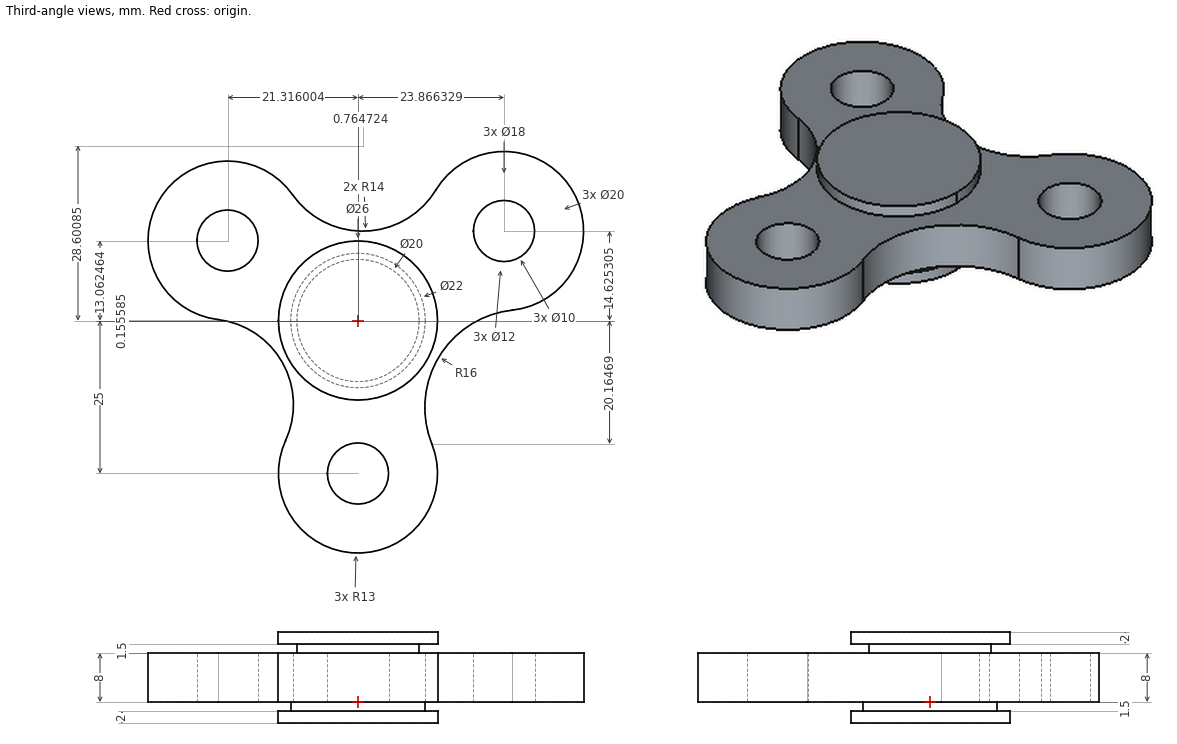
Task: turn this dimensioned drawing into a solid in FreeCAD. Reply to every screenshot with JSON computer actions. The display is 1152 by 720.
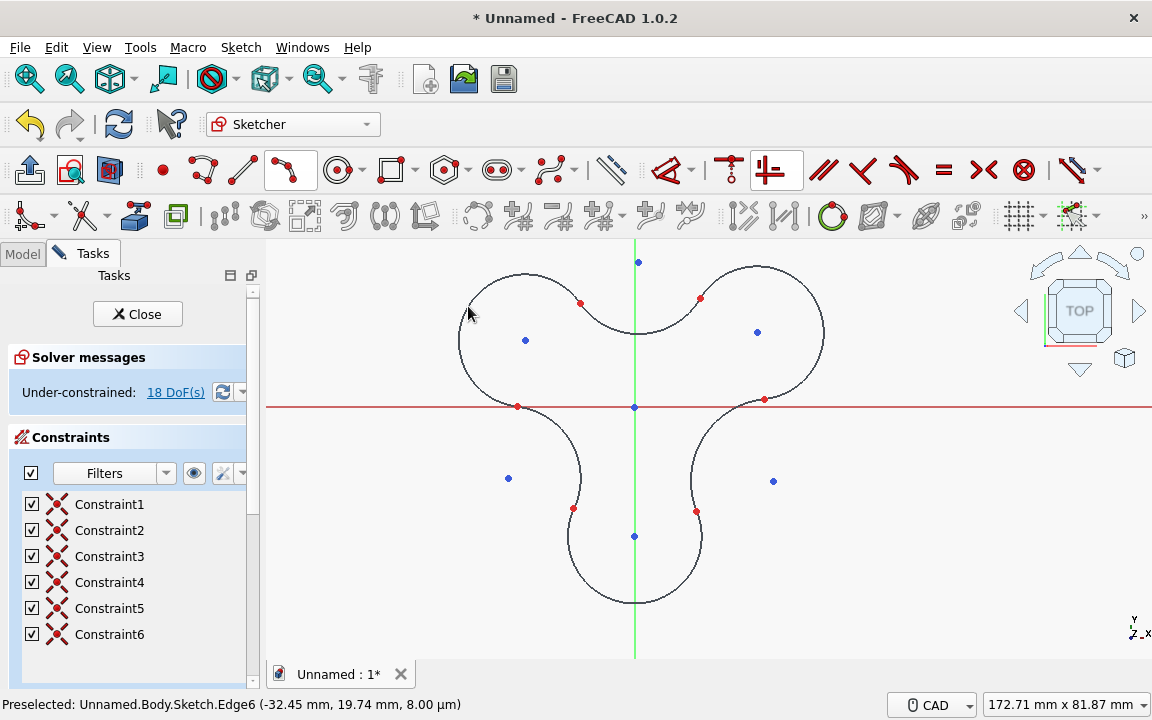
{"action": "left_click", "coordinate": [580, 469]}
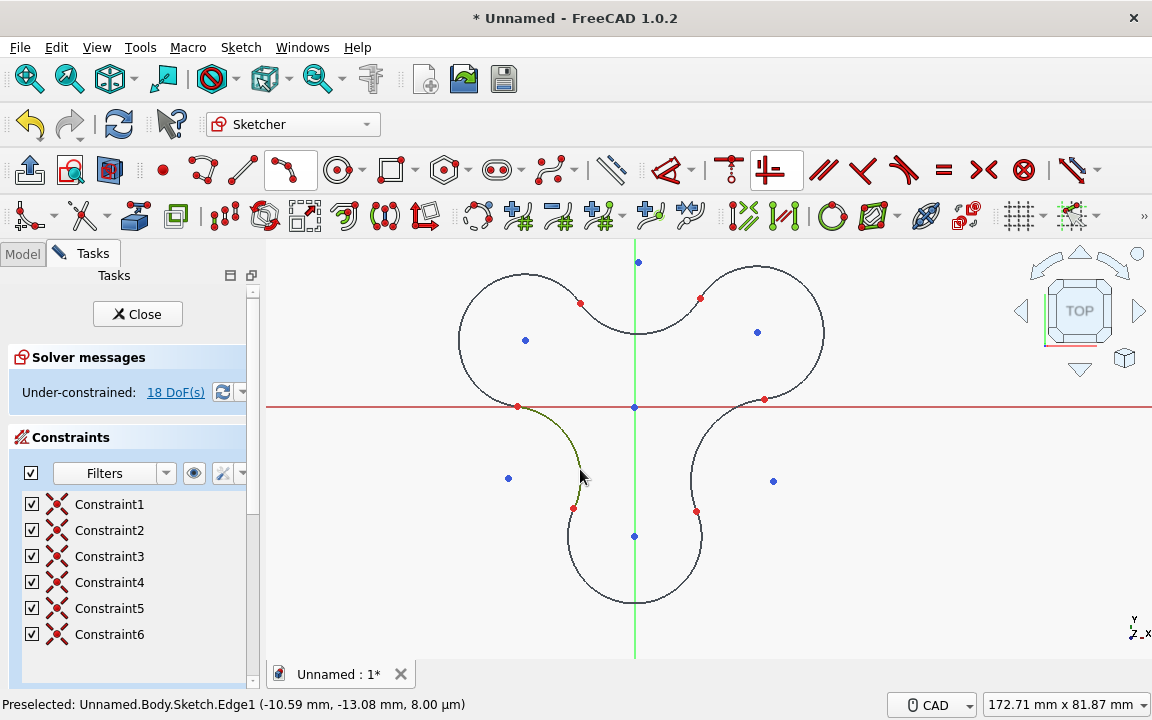
{"action": "left_click", "coordinate": [586, 583]}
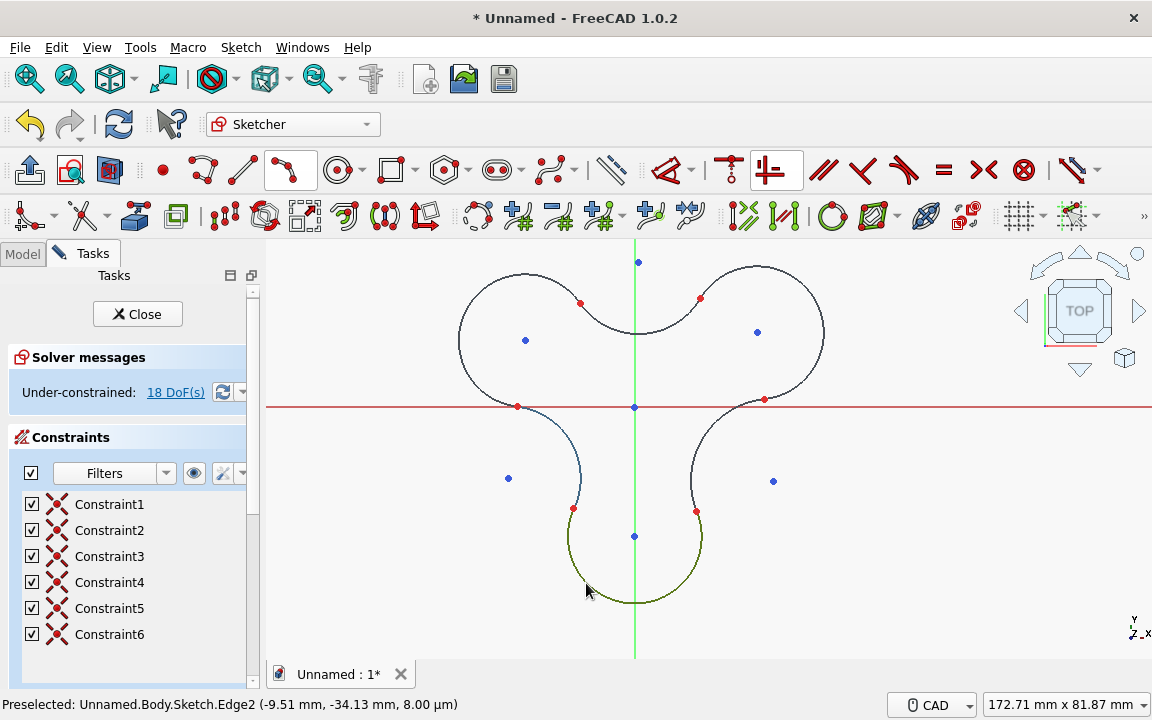
{"action": "left_click", "coordinate": [904, 170]}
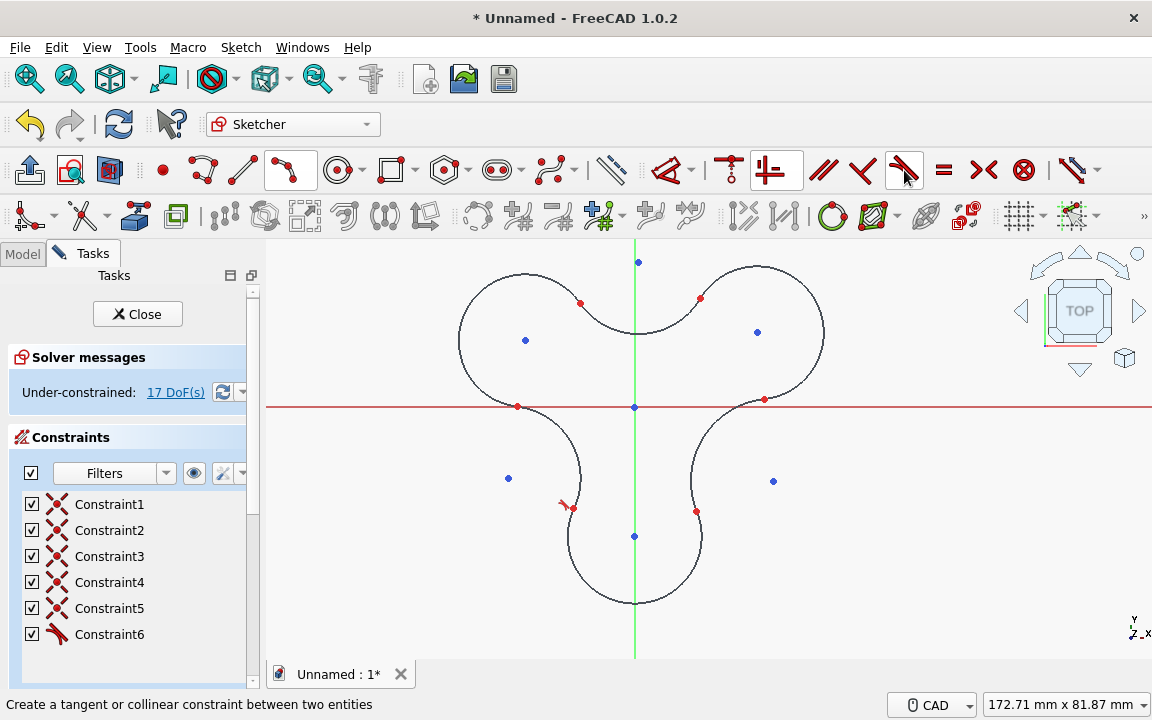
{"action": "left_click", "coordinate": [580, 469]}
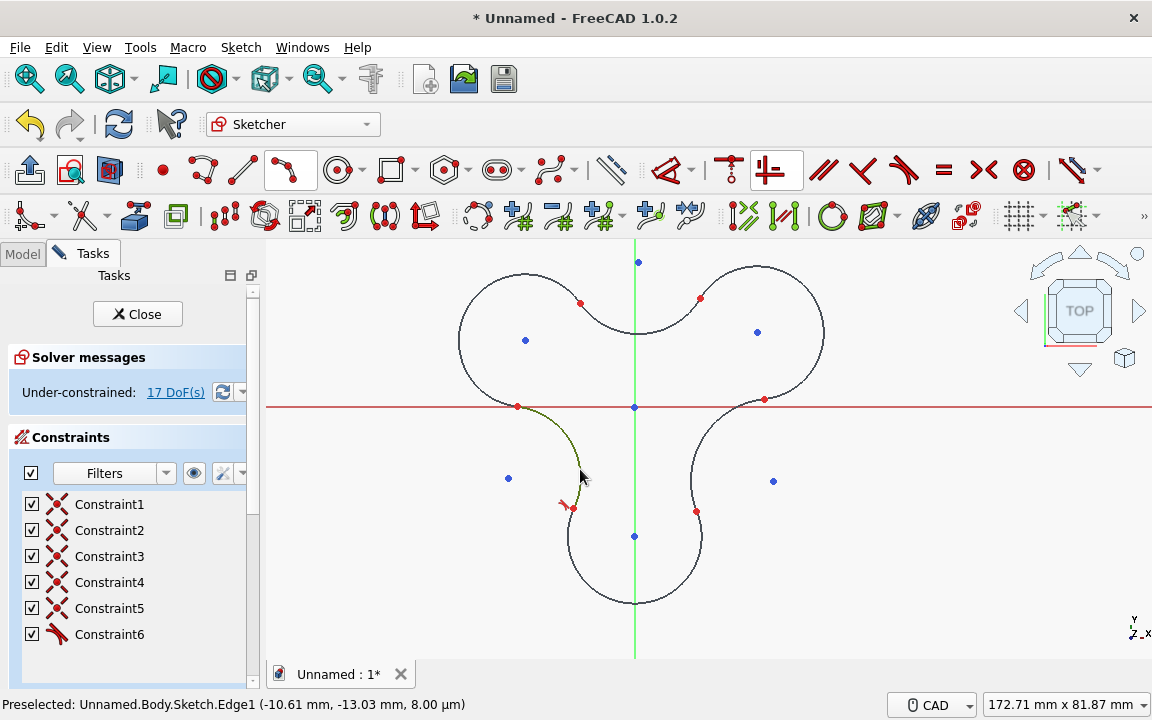
{"action": "left_click", "coordinate": [511, 276]}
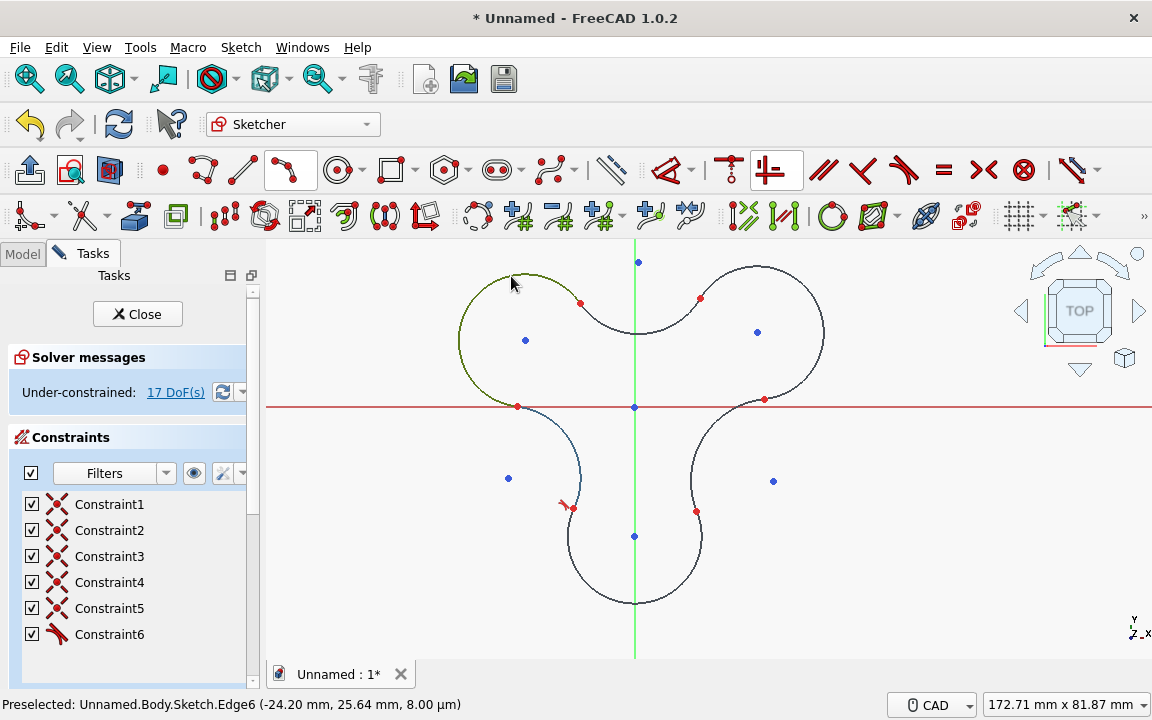
{"action": "left_click", "coordinate": [904, 170]}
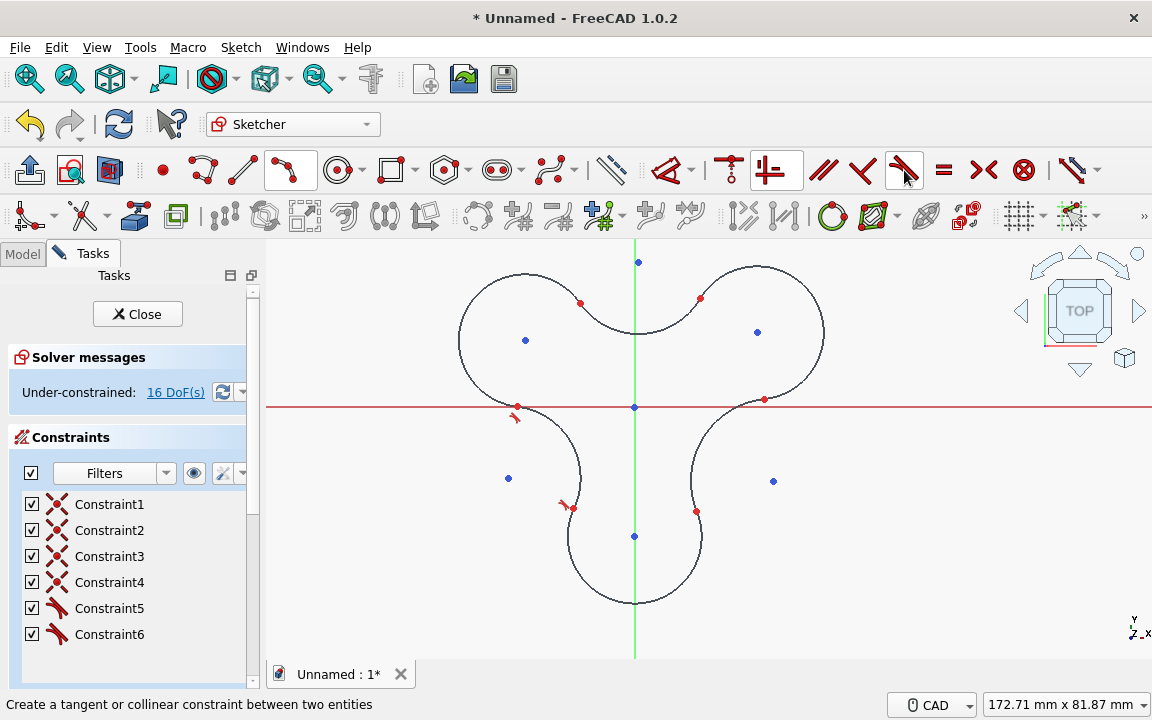
{"action": "left_click", "coordinate": [586, 582]}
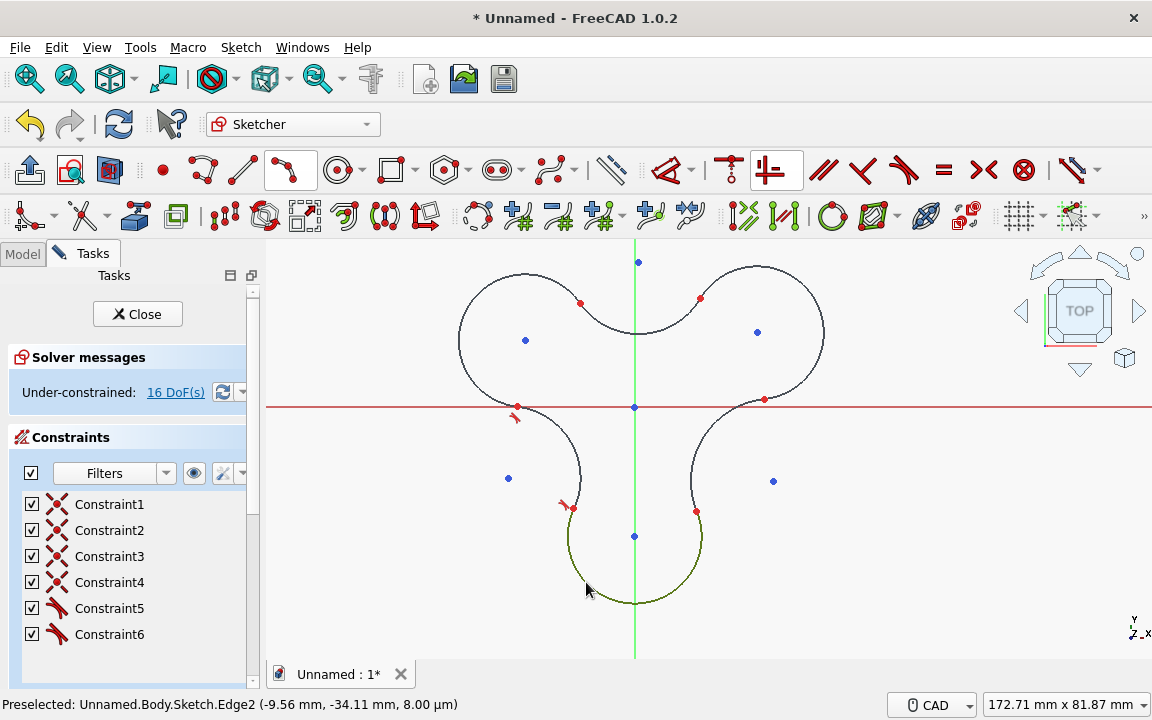
{"action": "left_click", "coordinate": [692, 467]}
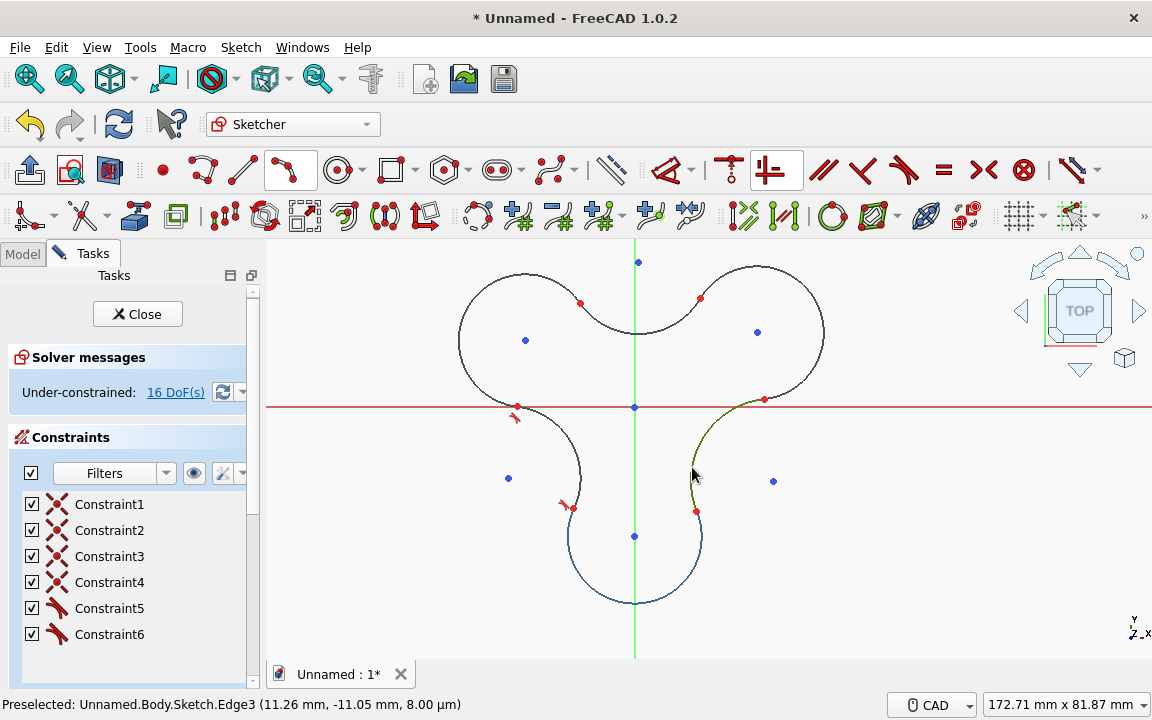
{"action": "left_click", "coordinate": [904, 170]}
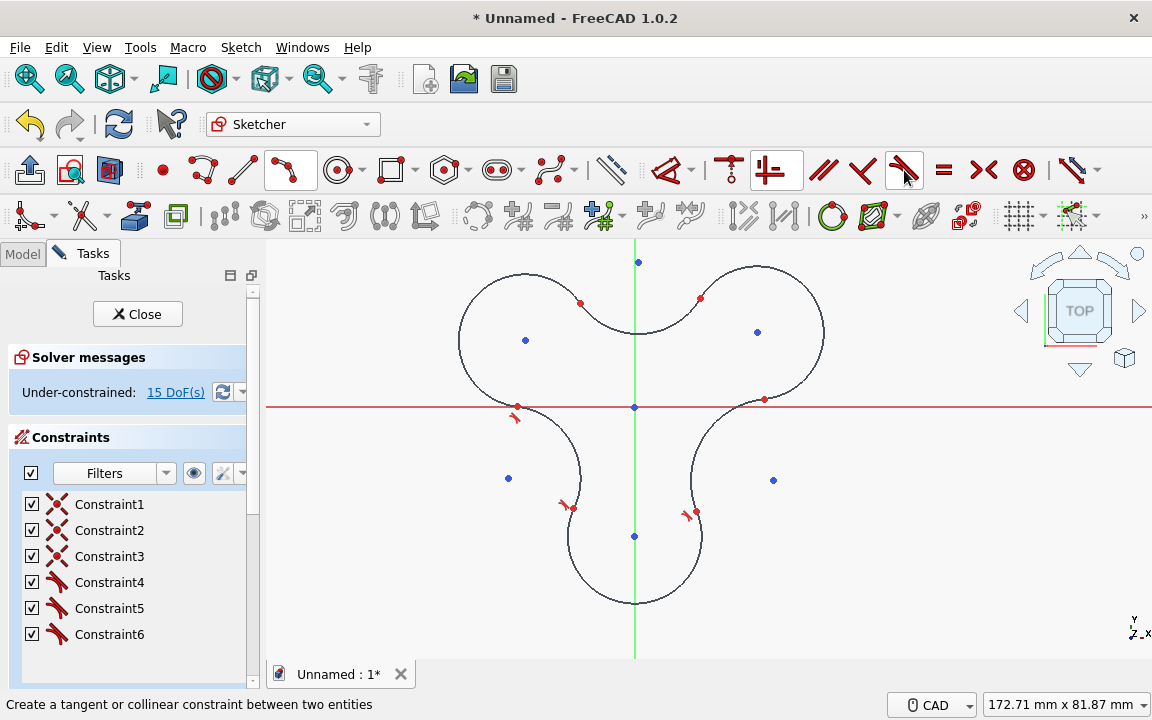
{"action": "left_click", "coordinate": [692, 467]}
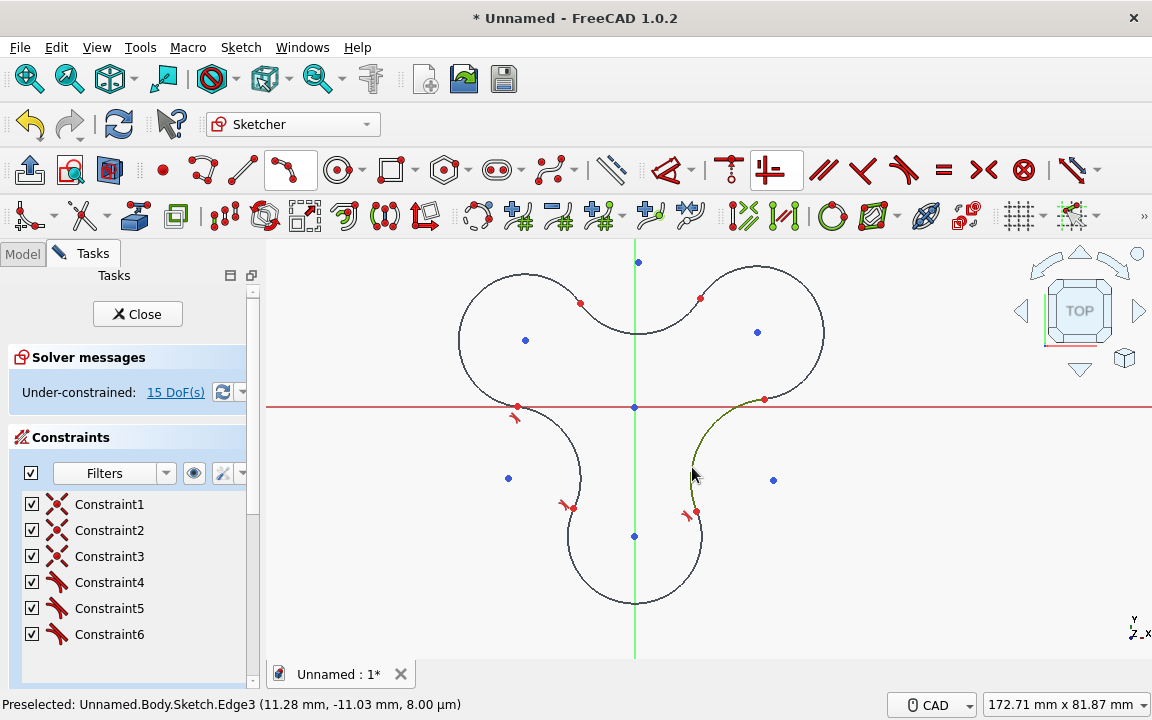
{"action": "left_click", "coordinate": [822, 349]}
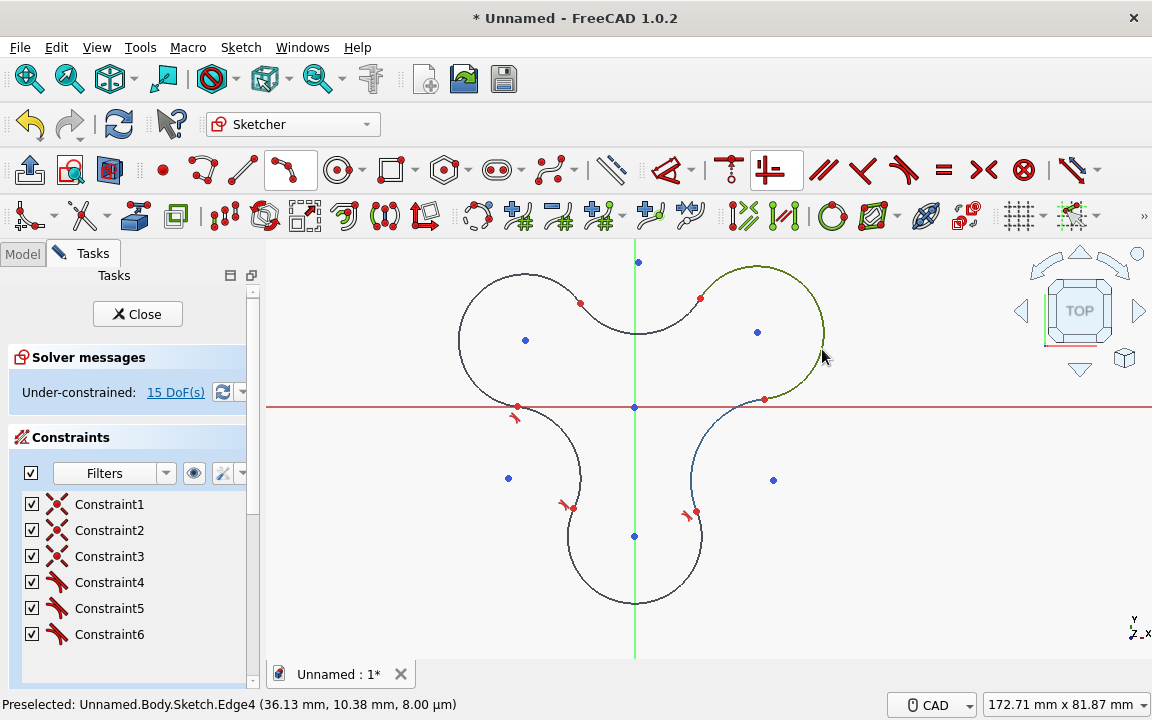
{"action": "left_click", "coordinate": [904, 170]}